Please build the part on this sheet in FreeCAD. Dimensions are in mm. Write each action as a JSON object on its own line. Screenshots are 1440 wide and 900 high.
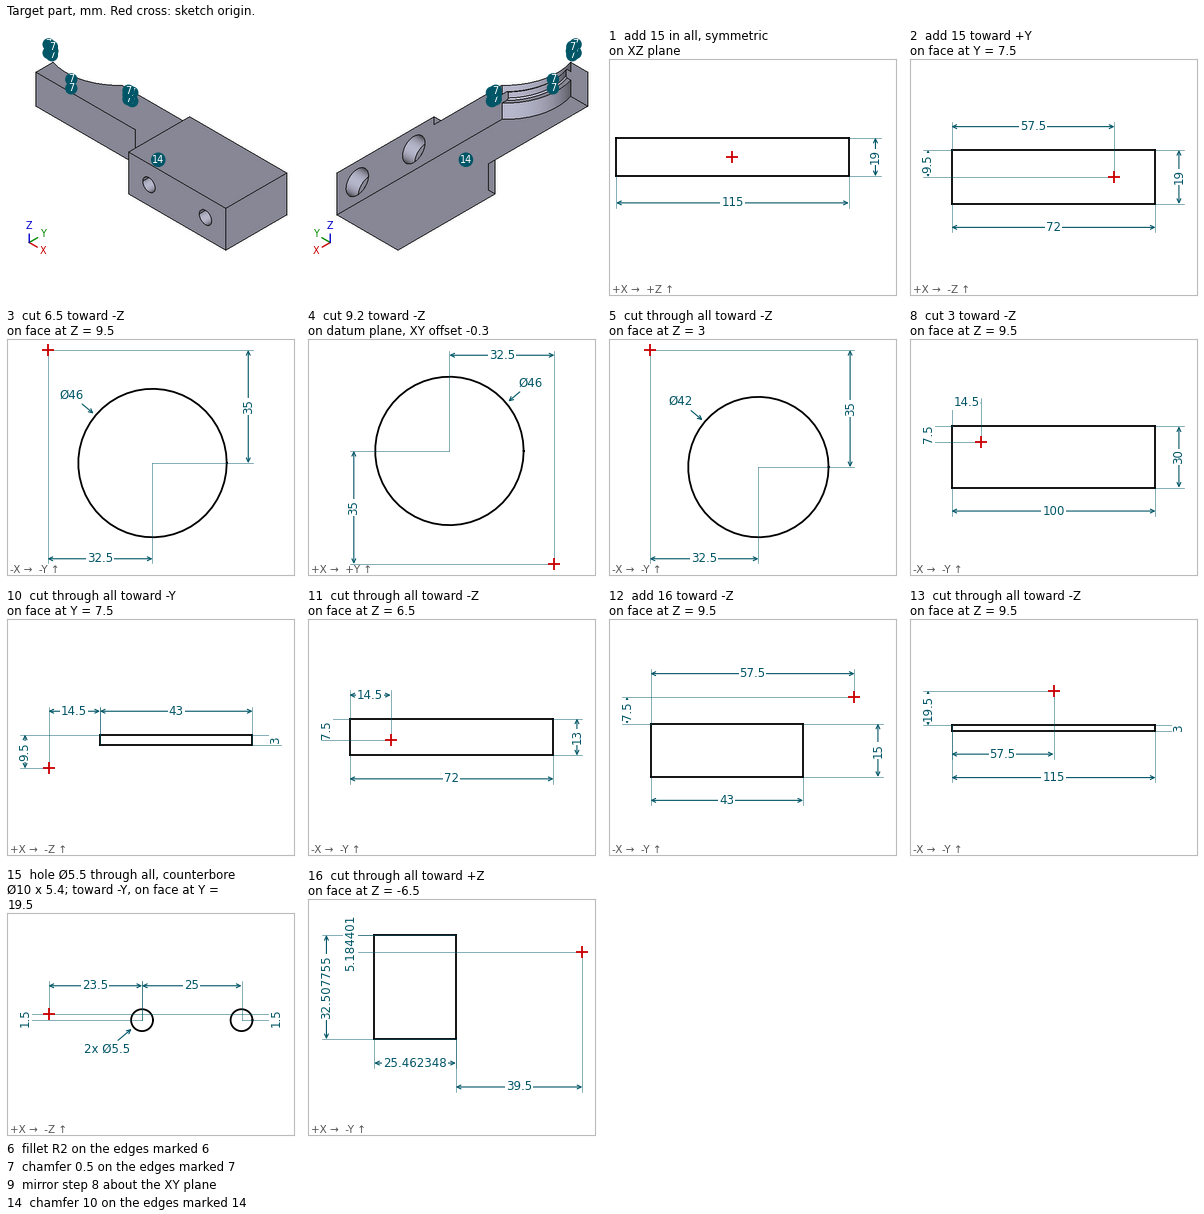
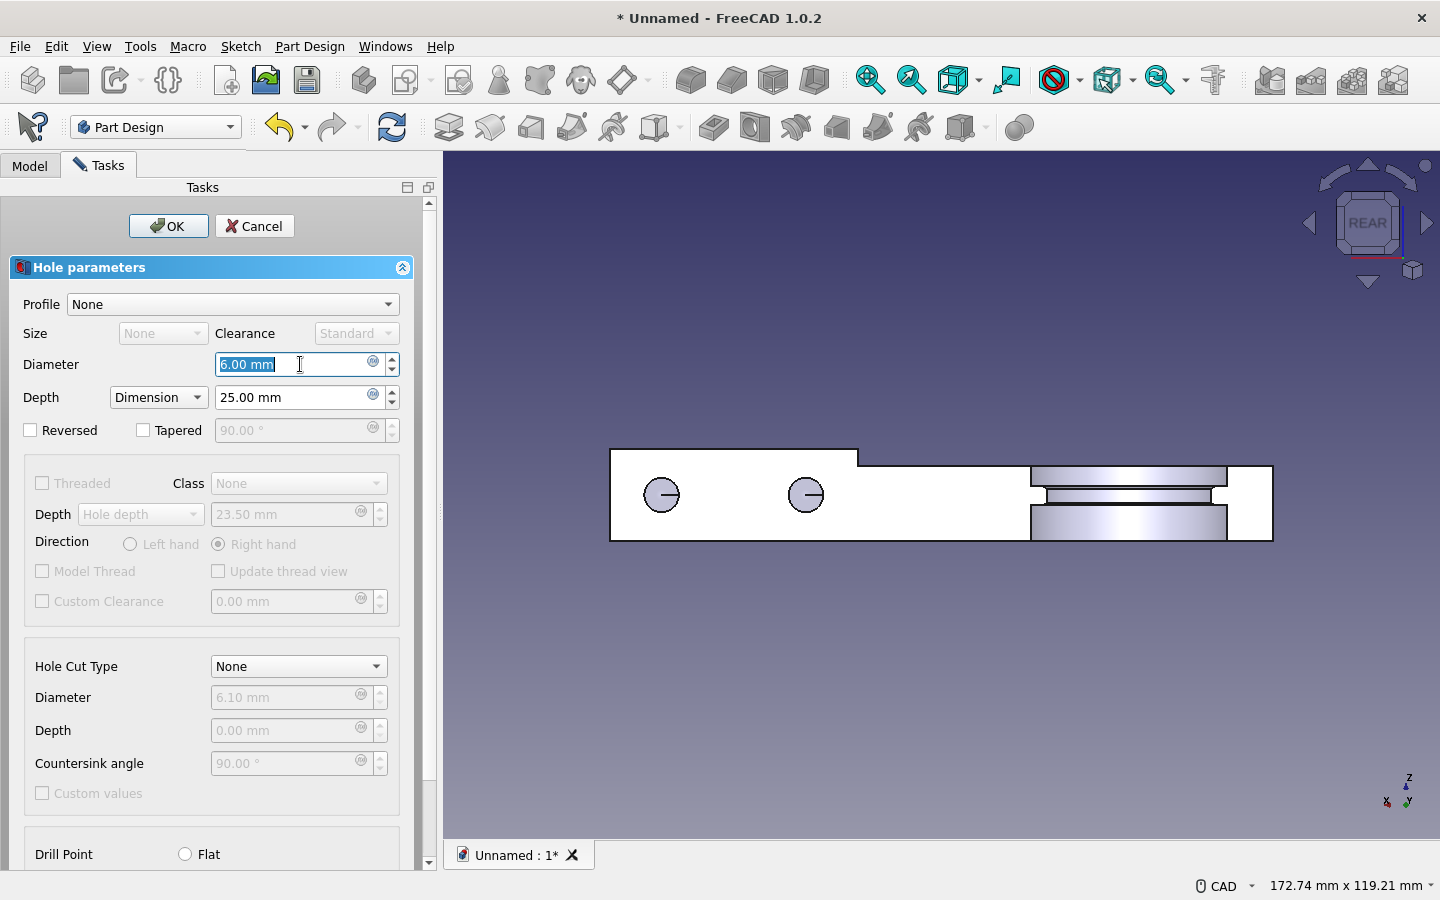
{"action": "type", "text": "5.5"}
{"action": "key", "text": "Tab"}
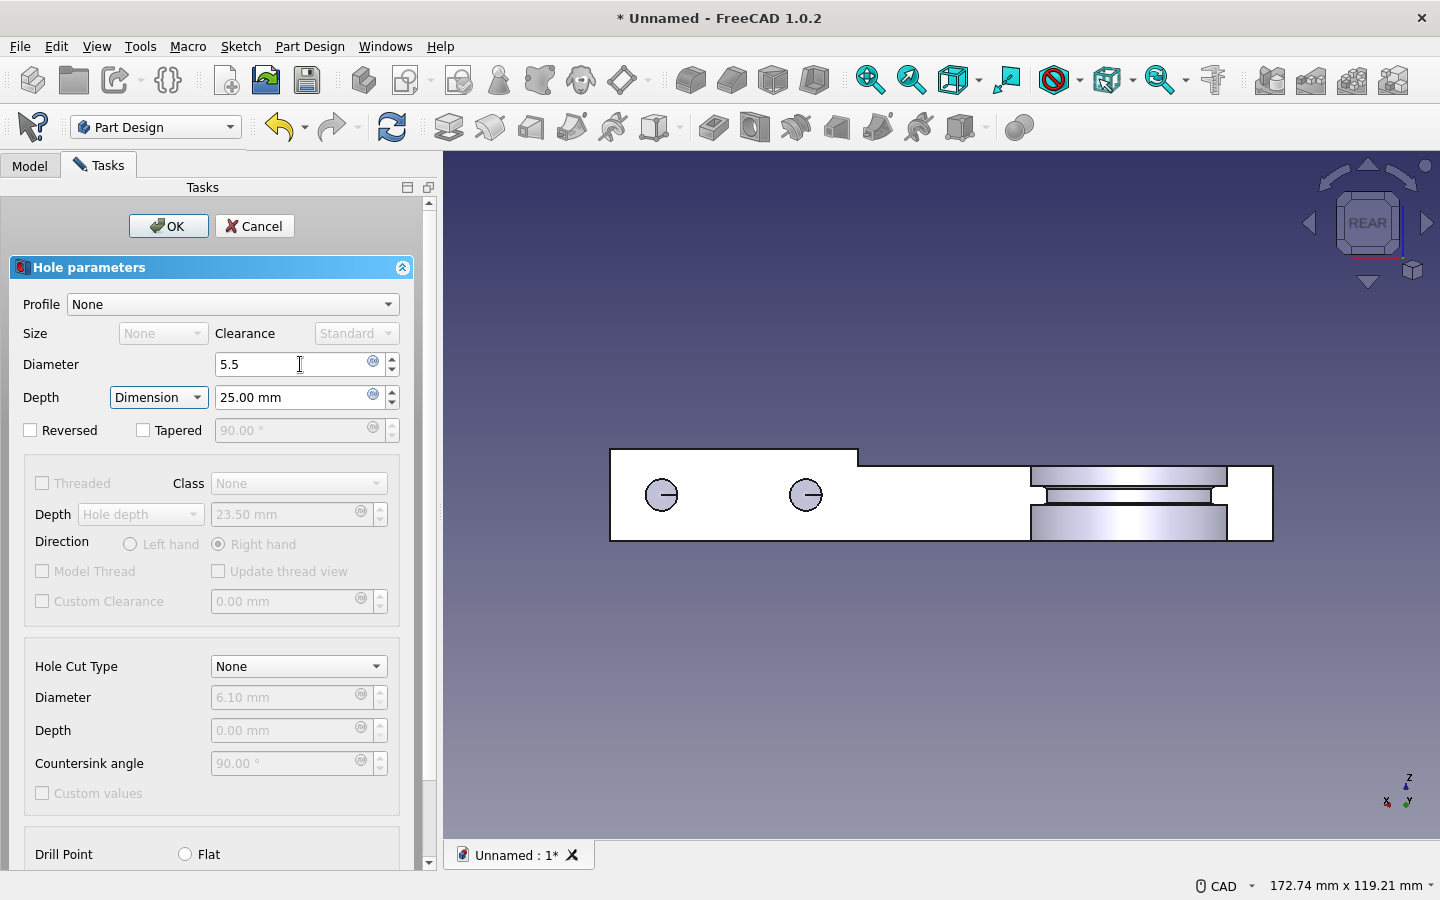
{"action": "left_click", "coordinate": [160, 398]}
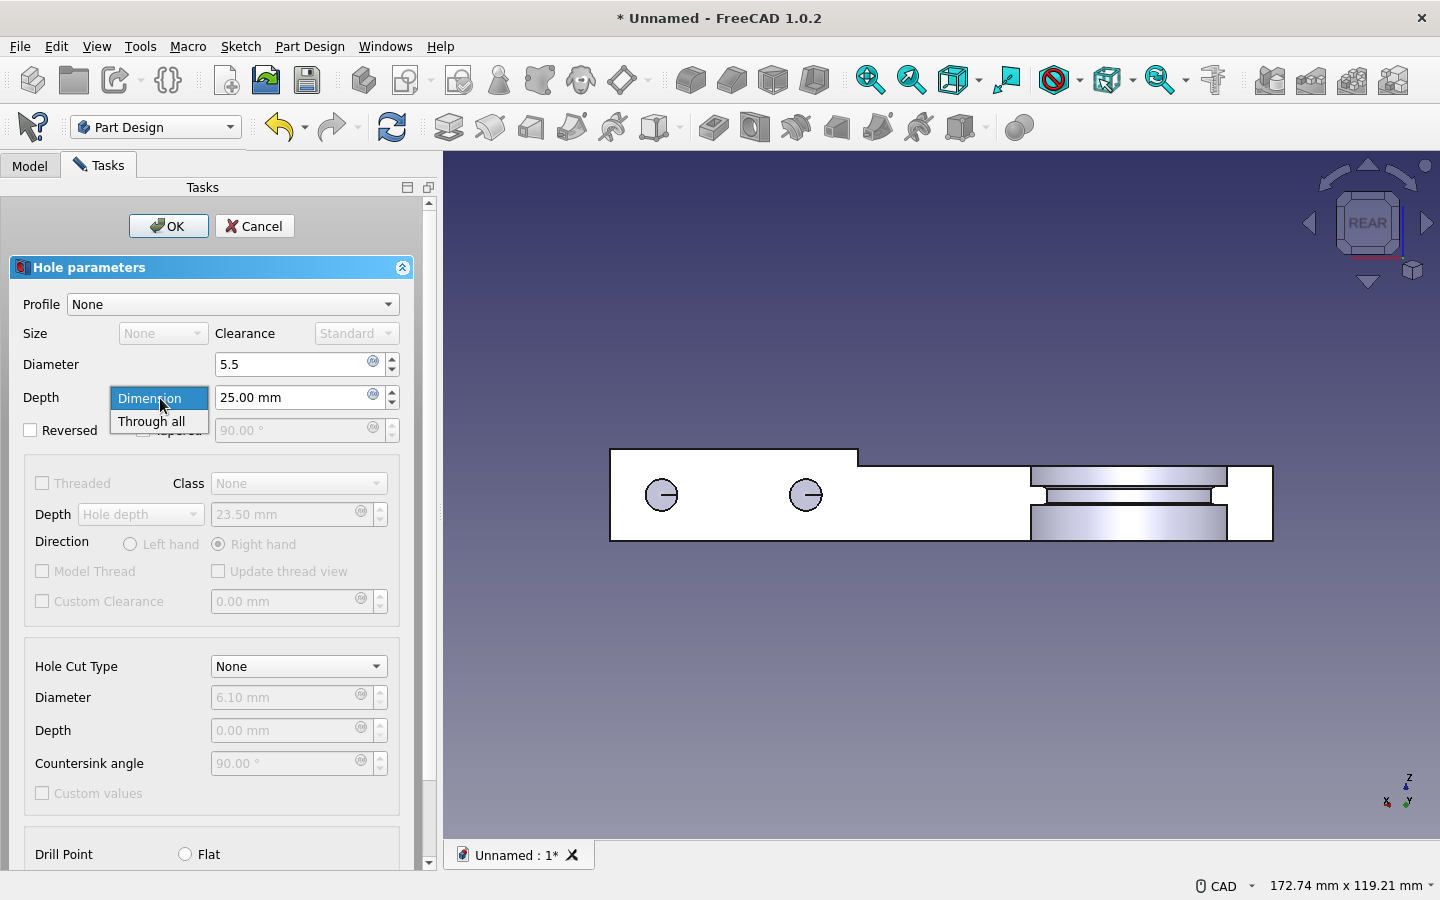
{"action": "left_click", "coordinate": [158, 422]}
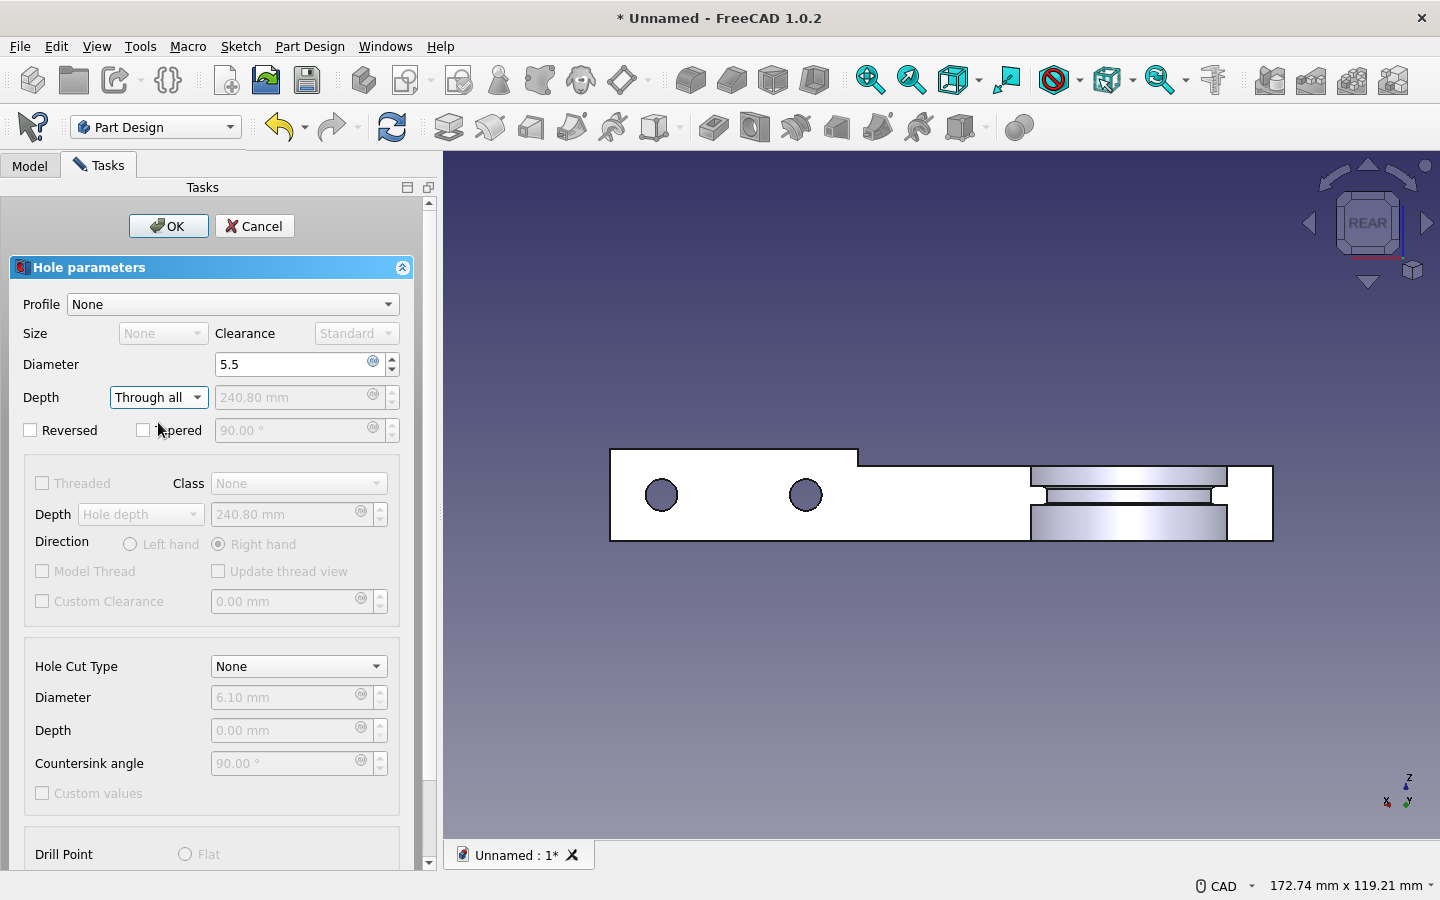
{"action": "left_click", "coordinate": [300, 666]}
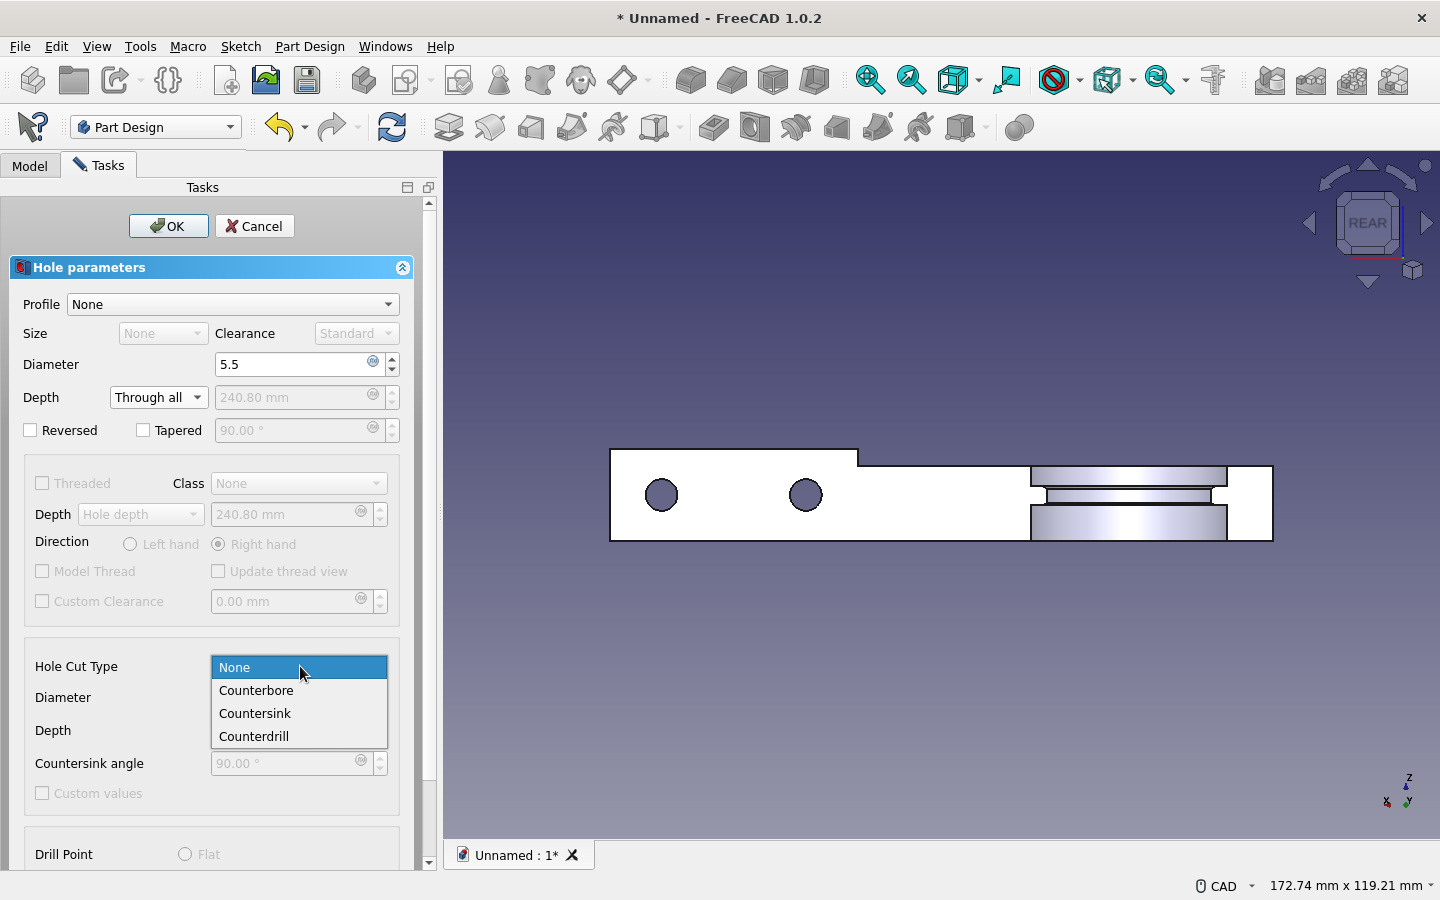
{"action": "left_click", "coordinate": [298, 690]}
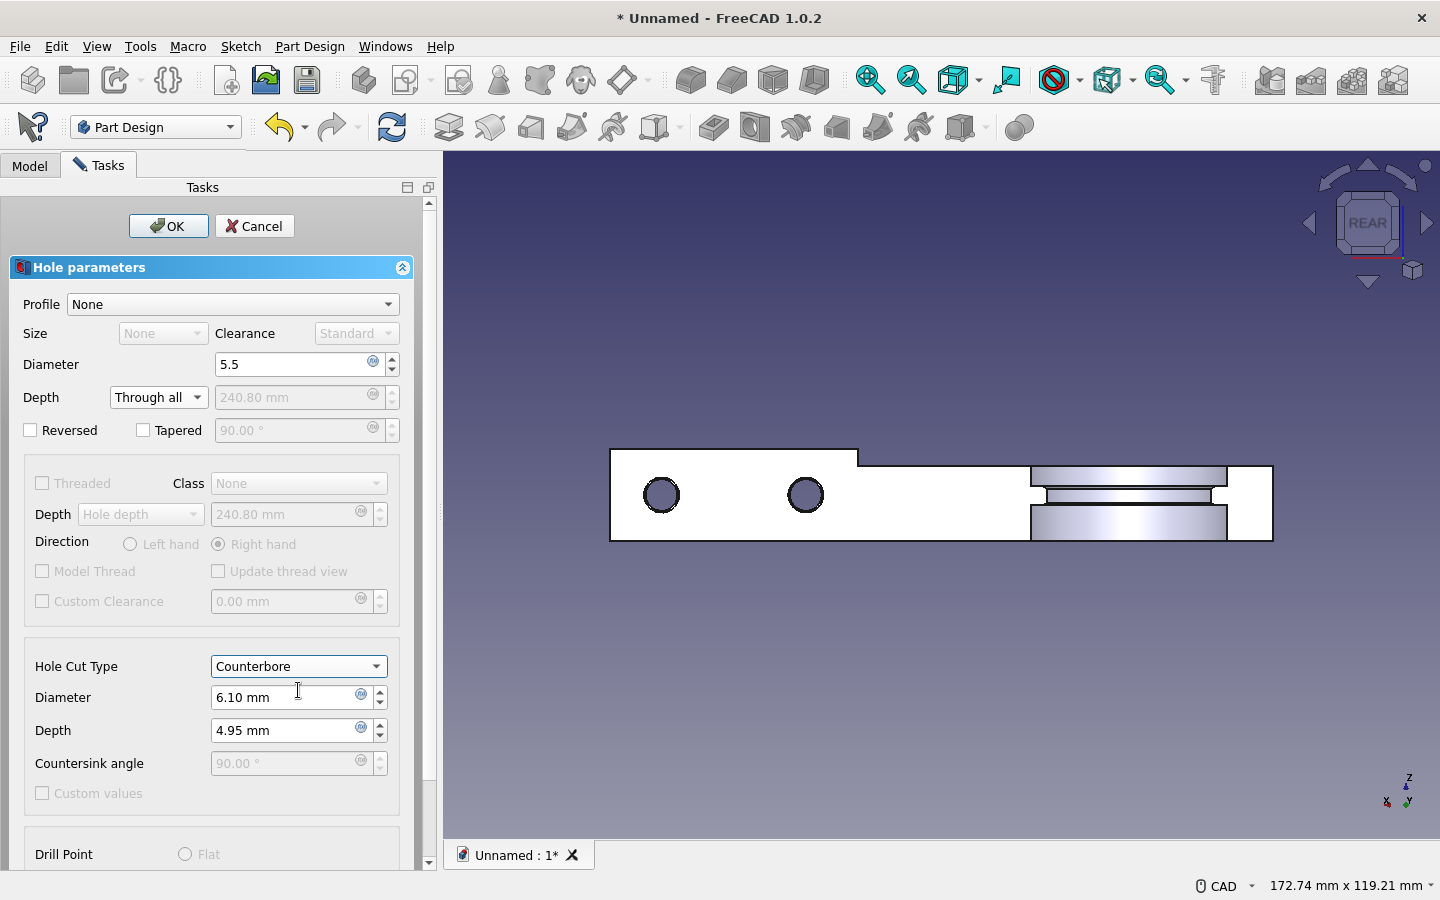
{"action": "triple_click", "coordinate": [292, 698]}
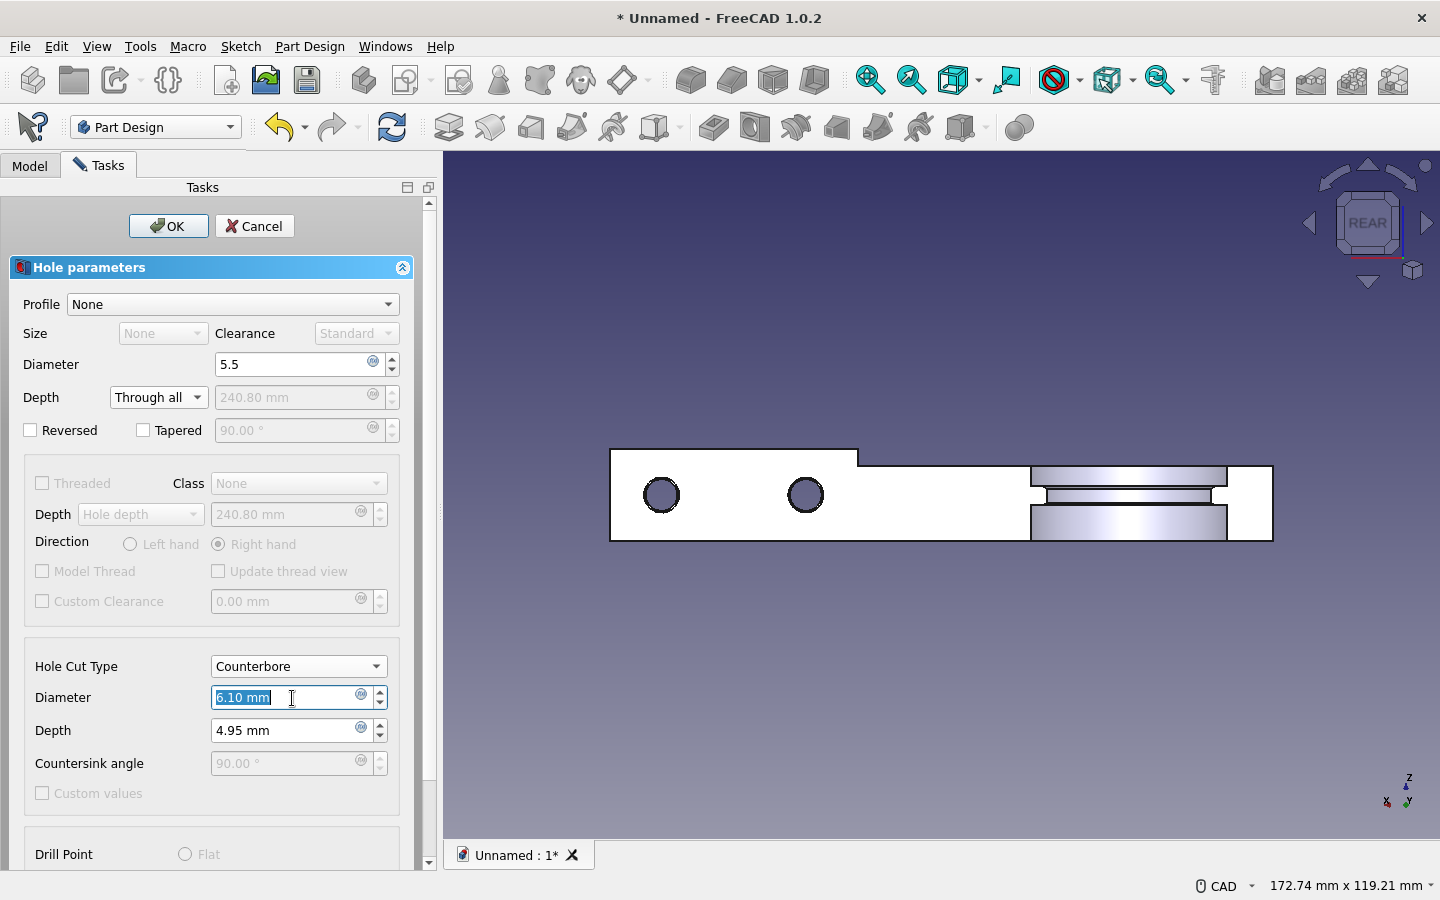
{"action": "type", "text": "10"}
{"action": "key", "text": "Tab"}